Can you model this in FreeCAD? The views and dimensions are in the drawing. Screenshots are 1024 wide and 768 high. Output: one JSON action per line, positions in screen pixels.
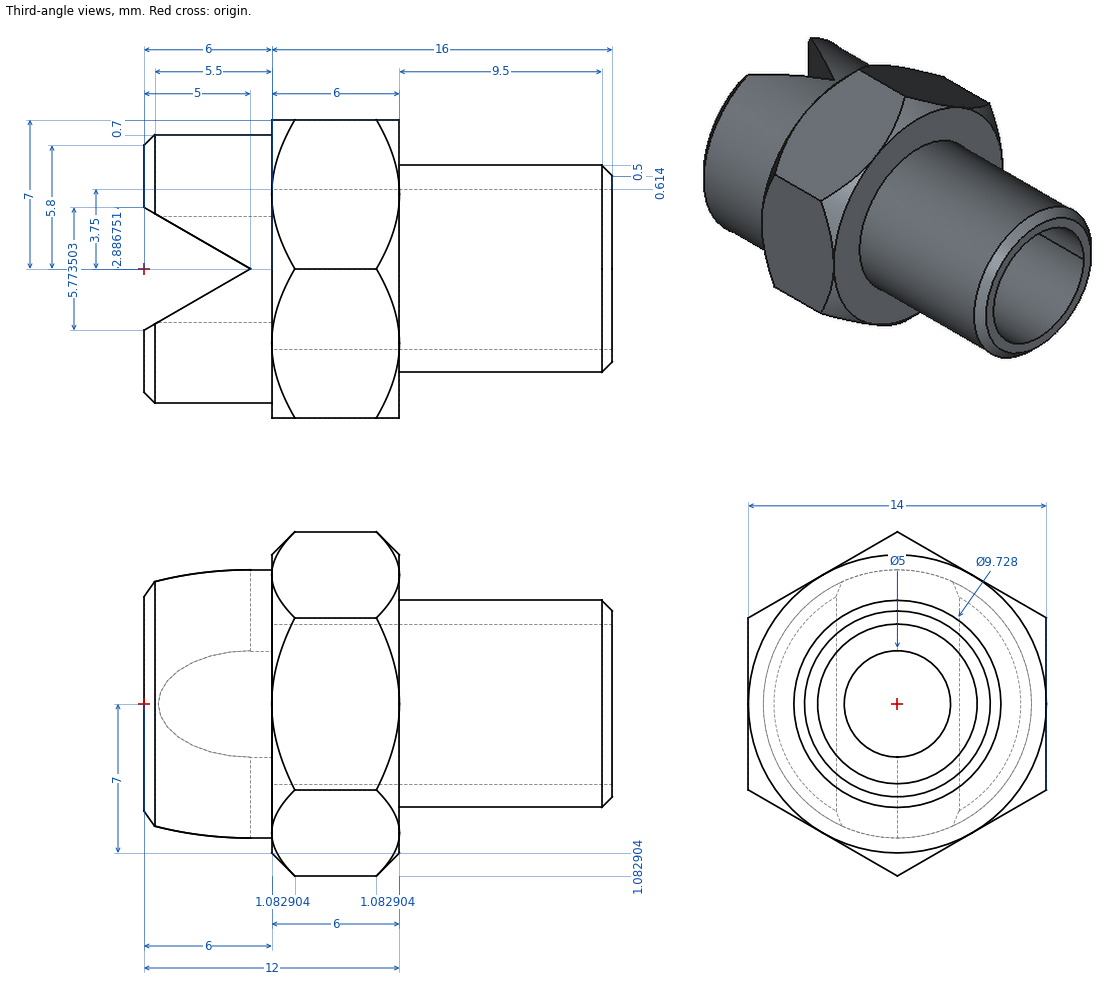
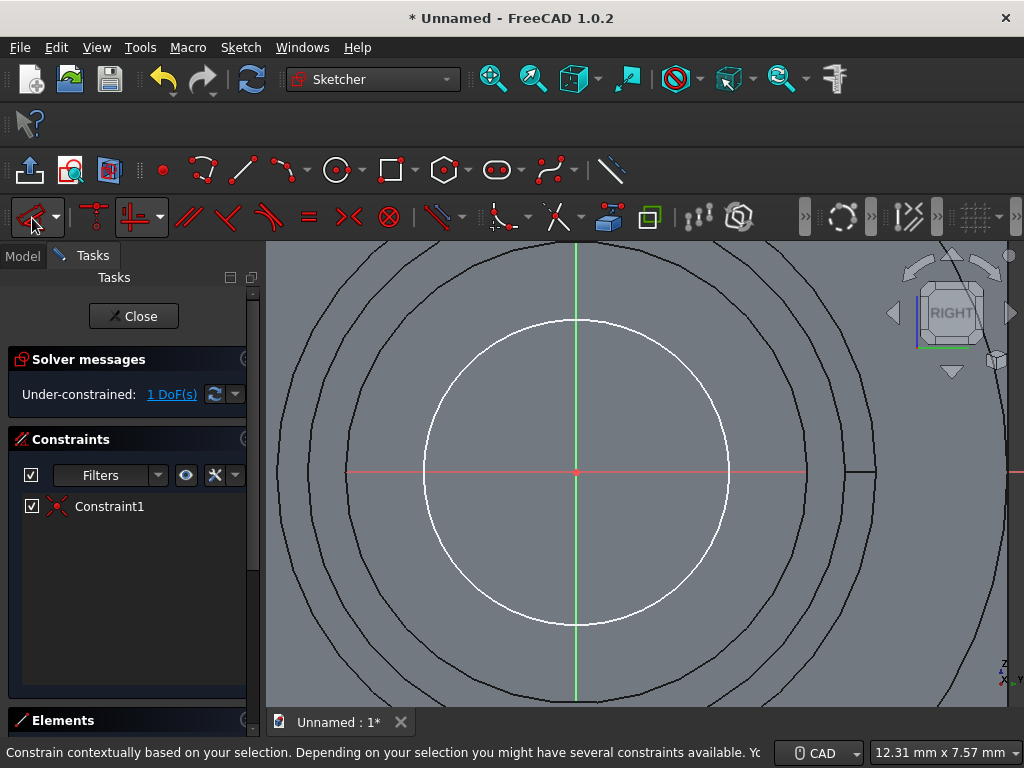
{"action": "left_click", "coordinate": [684, 364]}
{"action": "left_click", "coordinate": [707, 341]}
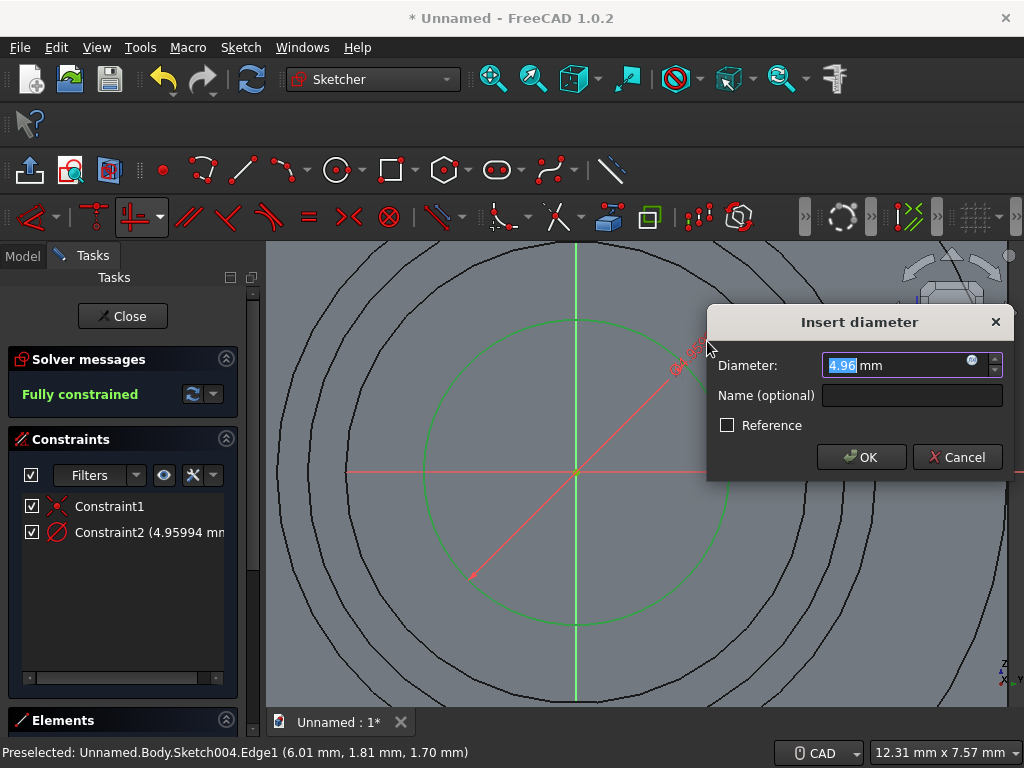
{"action": "type", "text": "5"}
{"action": "key", "text": "Return"}
{"action": "key", "text": "Escape"}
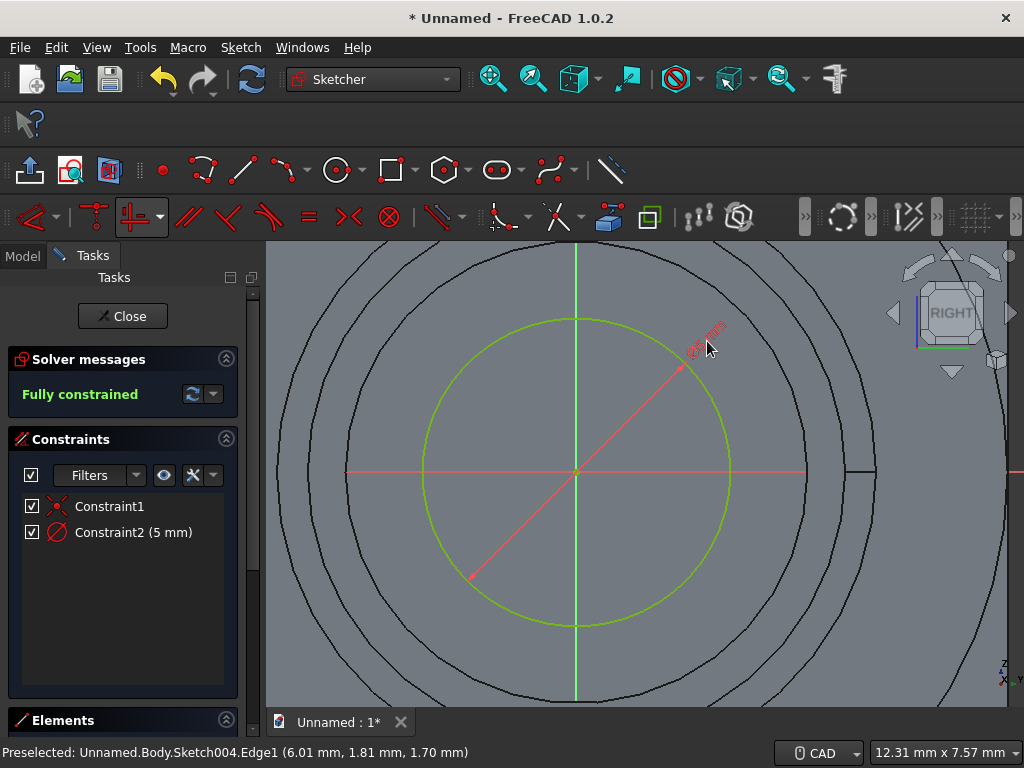
{"action": "left_click", "coordinate": [123, 316]}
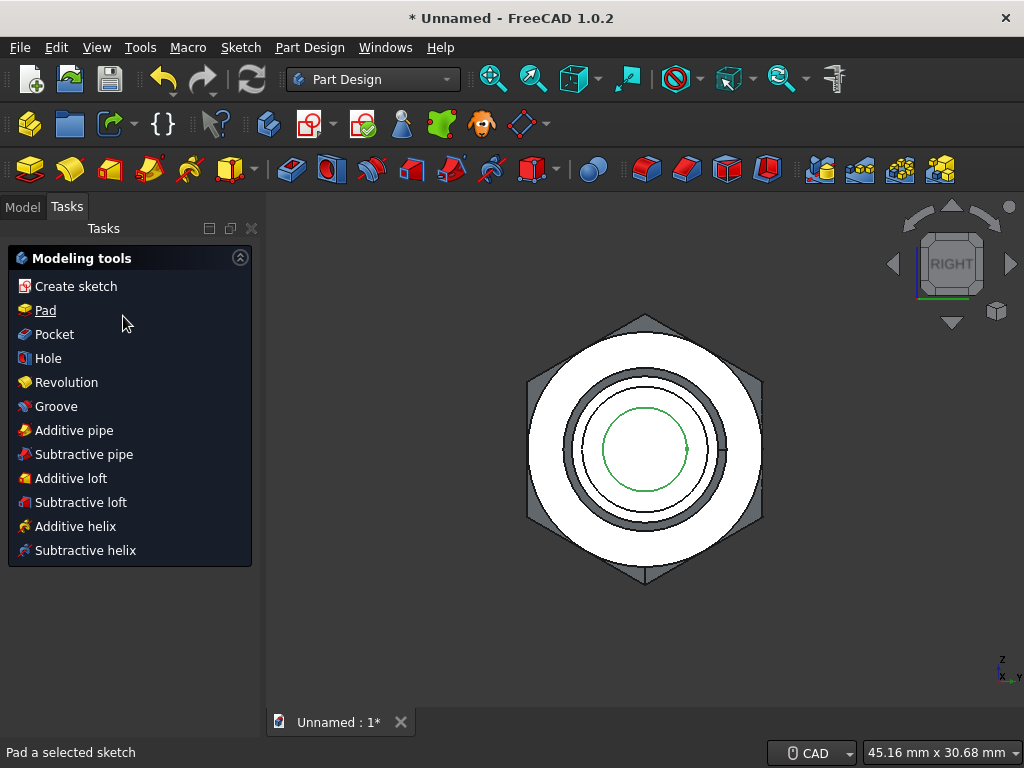
{"action": "left_click", "coordinate": [292, 170]}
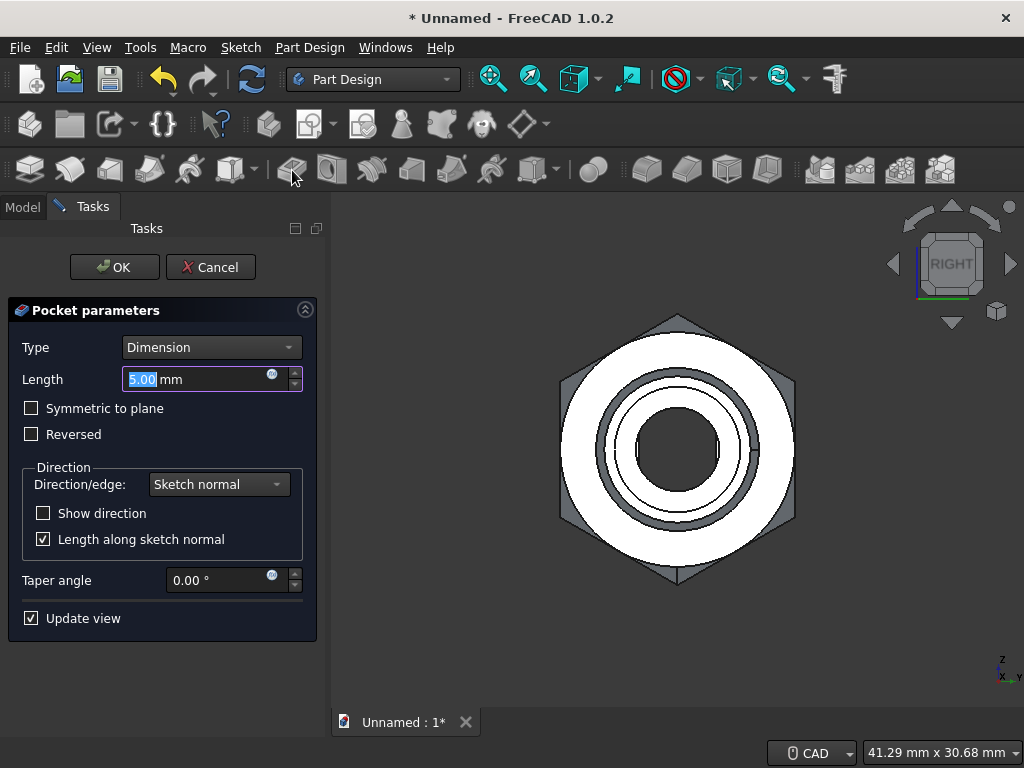
{"action": "left_click", "coordinate": [212, 348]}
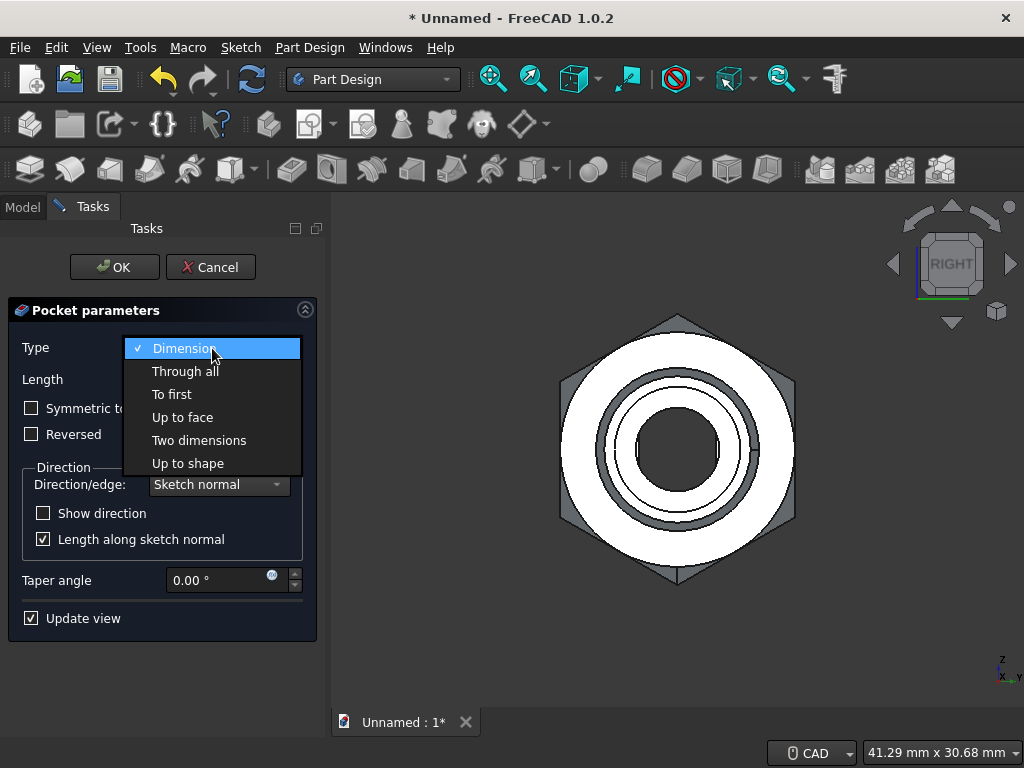
{"action": "left_click", "coordinate": [212, 372]}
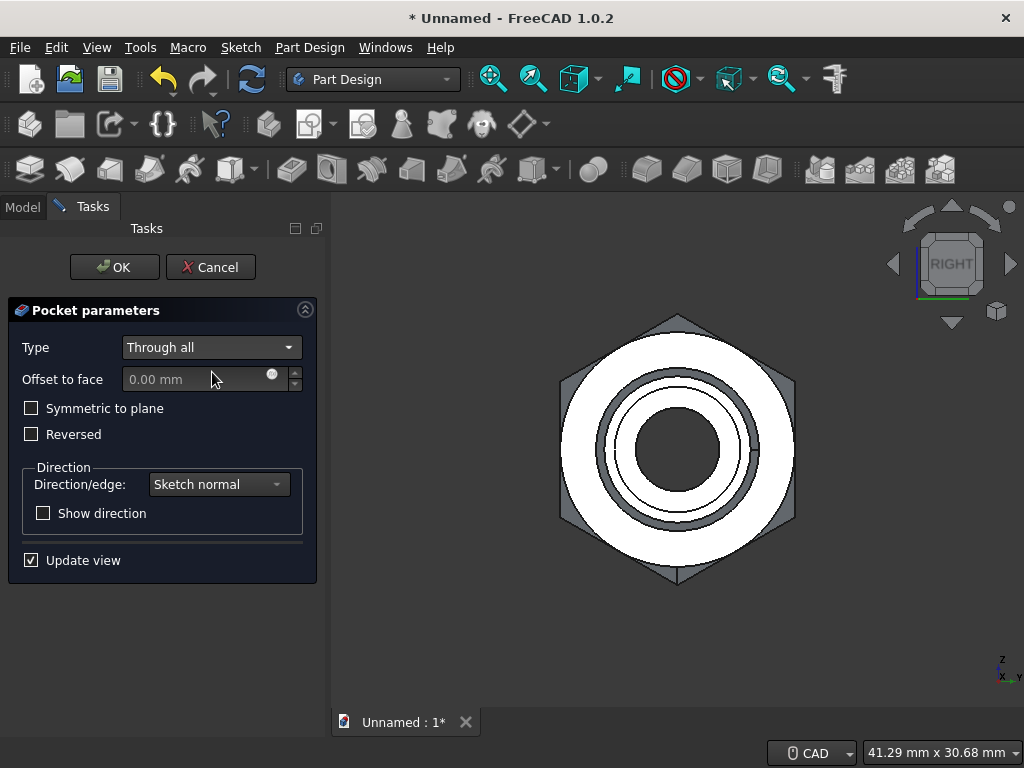
{"action": "left_click", "coordinate": [115, 267]}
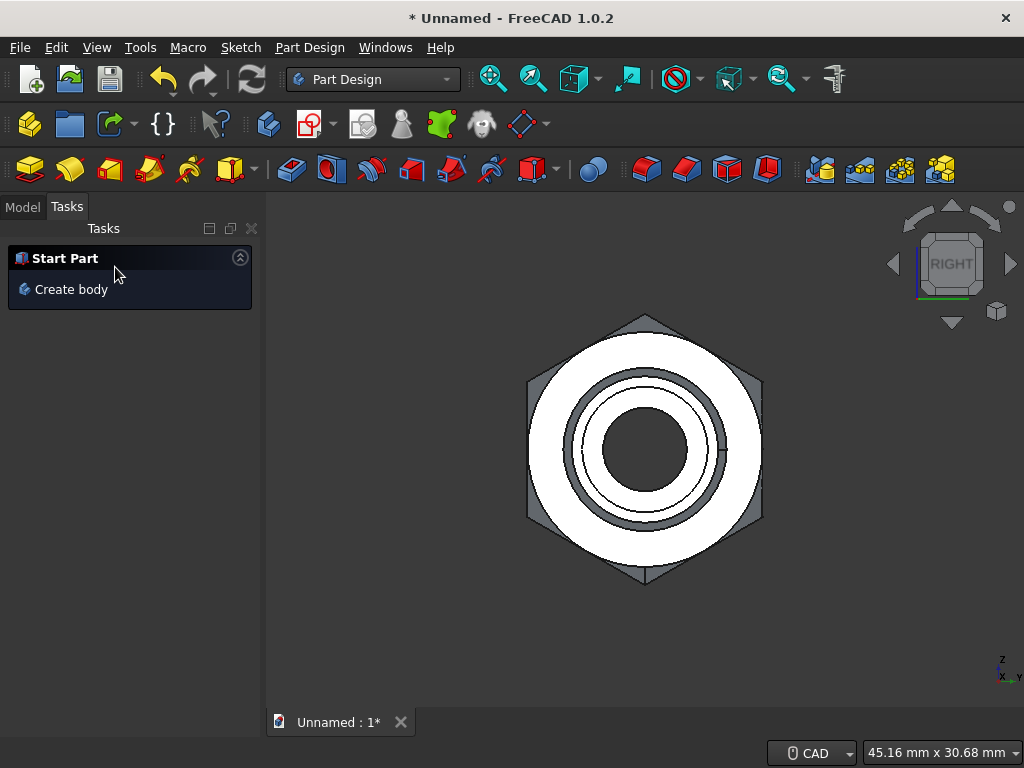
{"action": "key", "text": "0"}